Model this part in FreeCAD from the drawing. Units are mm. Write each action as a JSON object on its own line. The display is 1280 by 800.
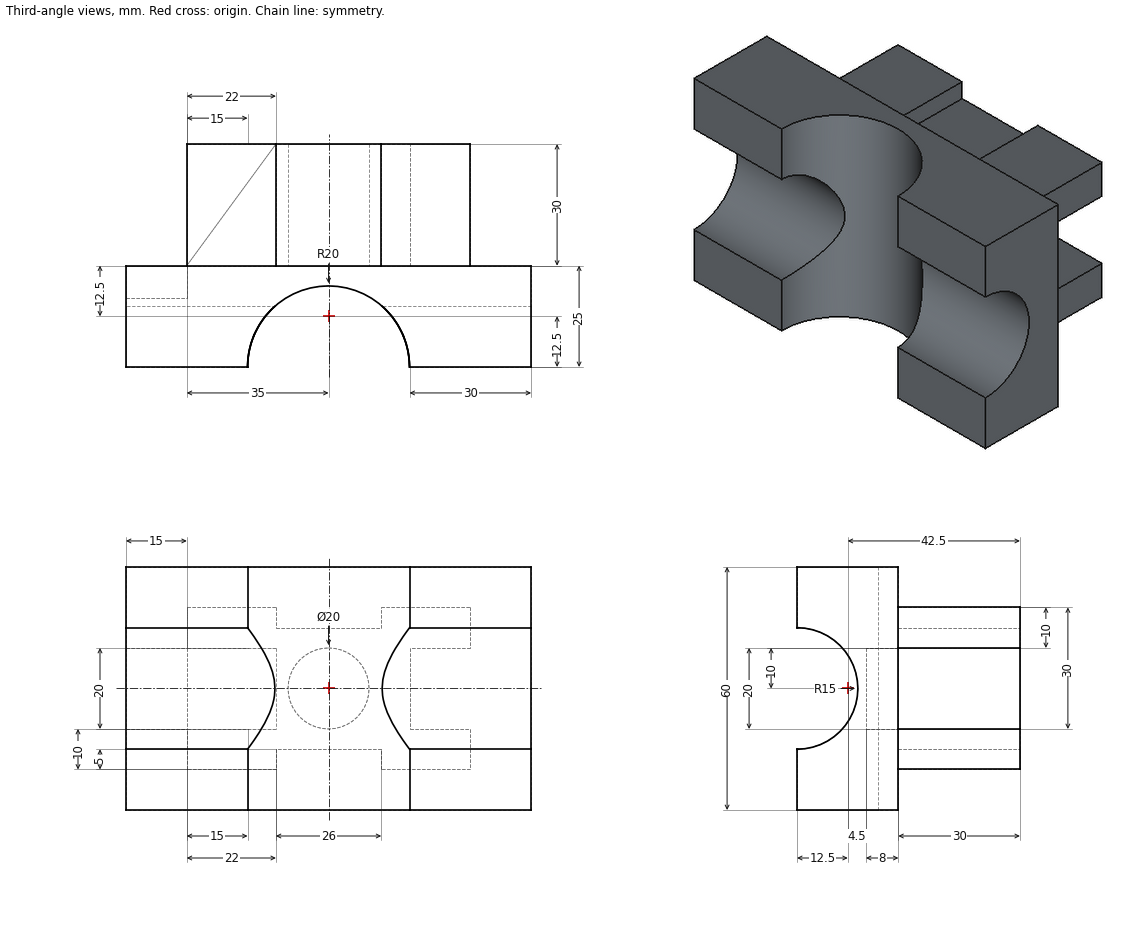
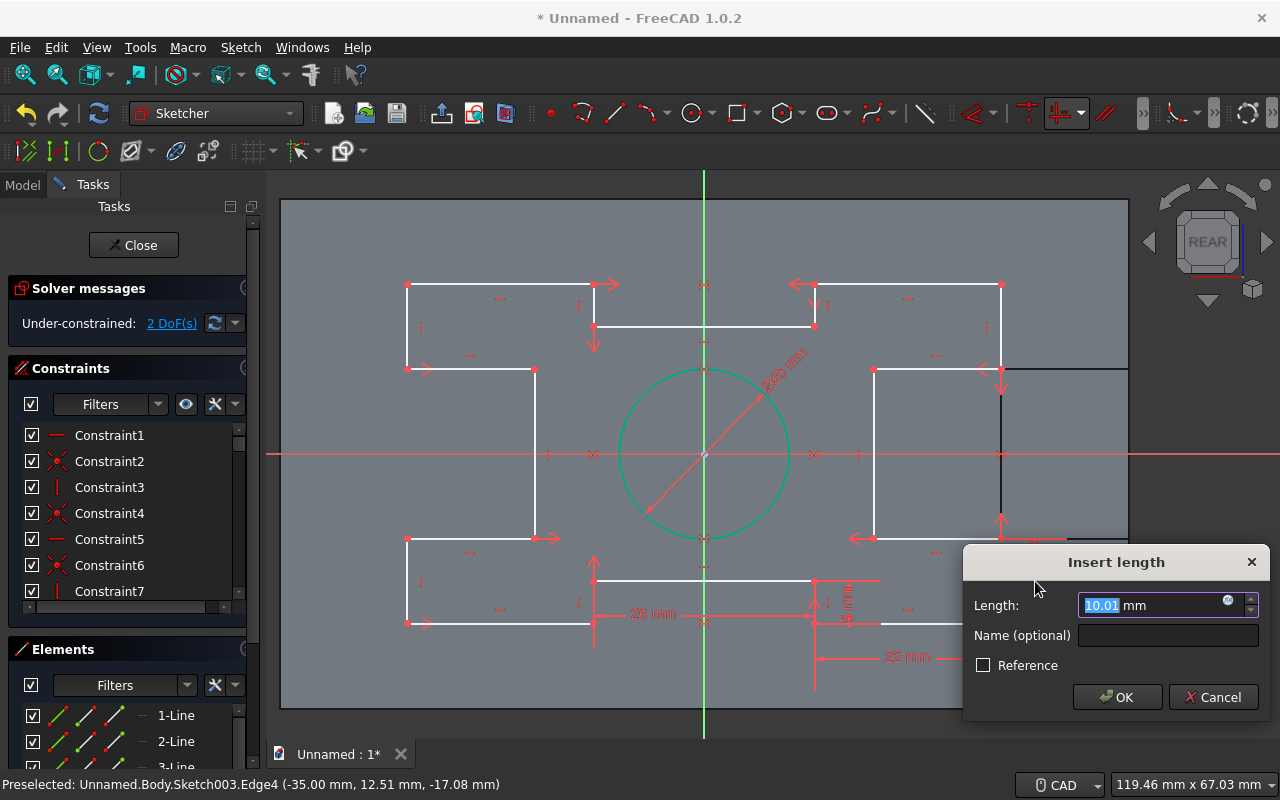
{"action": "type", "text": "10"}
{"action": "key", "text": "Return"}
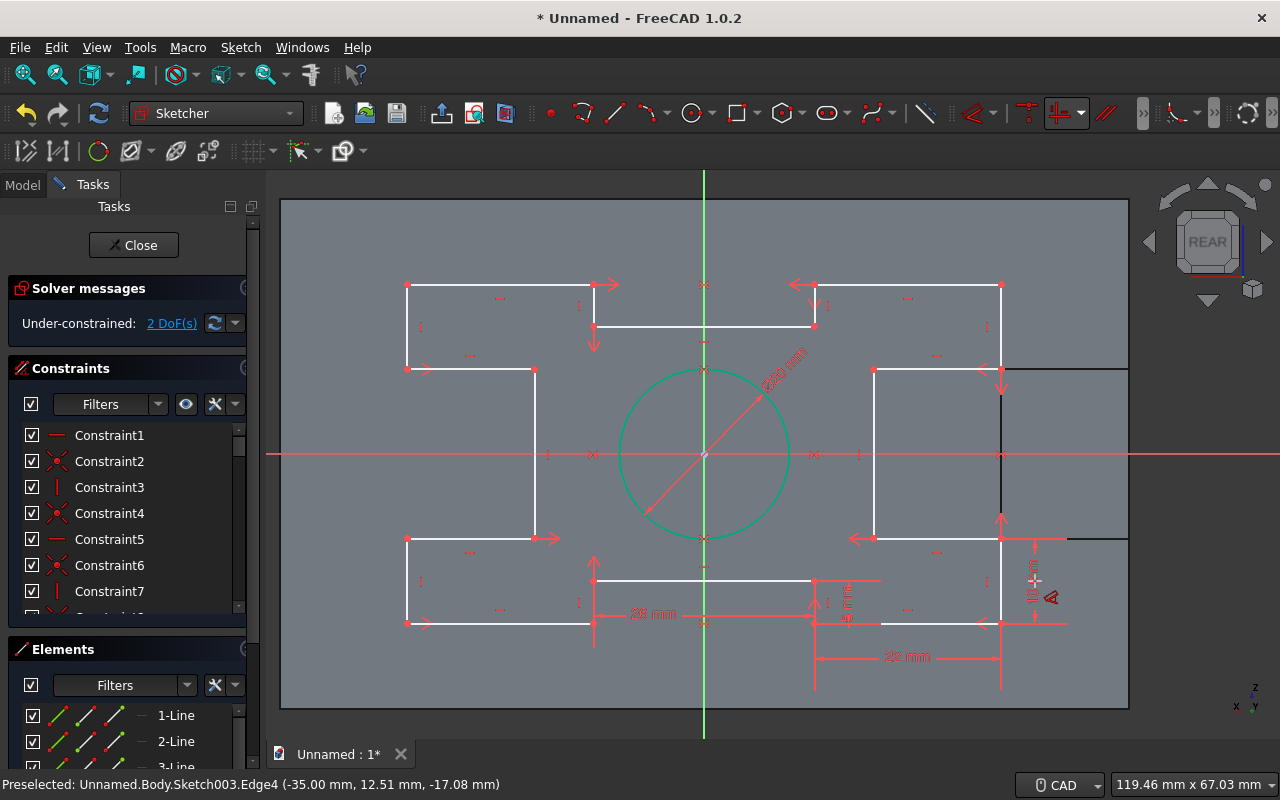
{"action": "left_click", "coordinate": [963, 539]}
{"action": "left_click", "coordinate": [938, 573]}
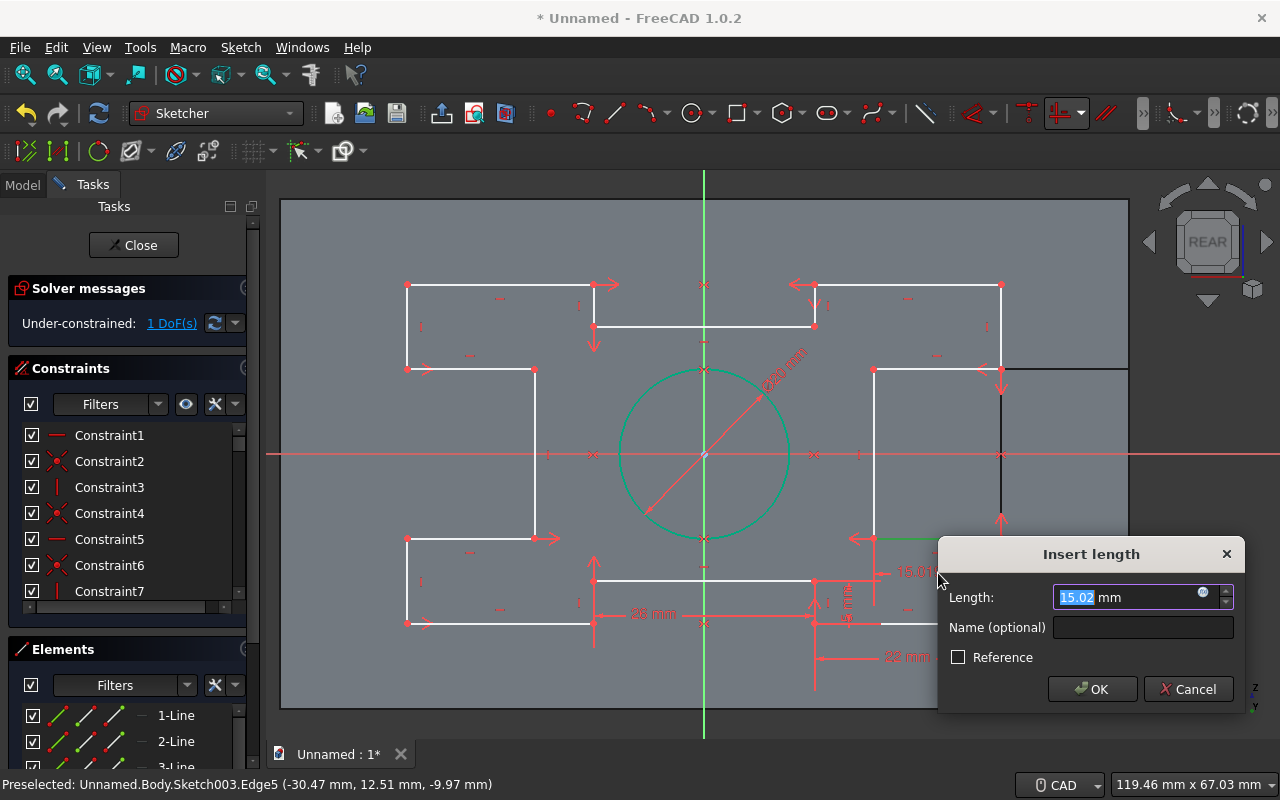
{"action": "type", "text": "15"}
{"action": "key", "text": "Return"}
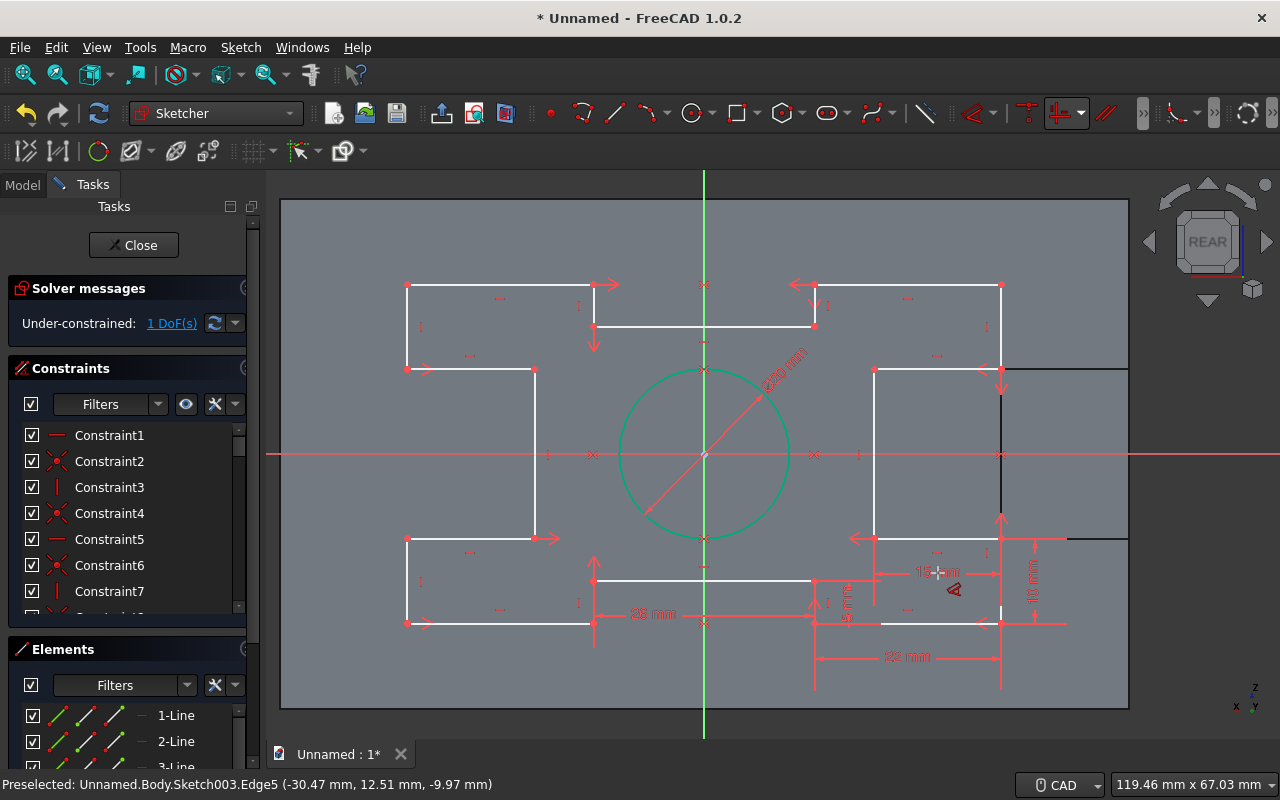
{"action": "left_click", "coordinate": [874, 488]}
{"action": "left_click", "coordinate": [908, 415]}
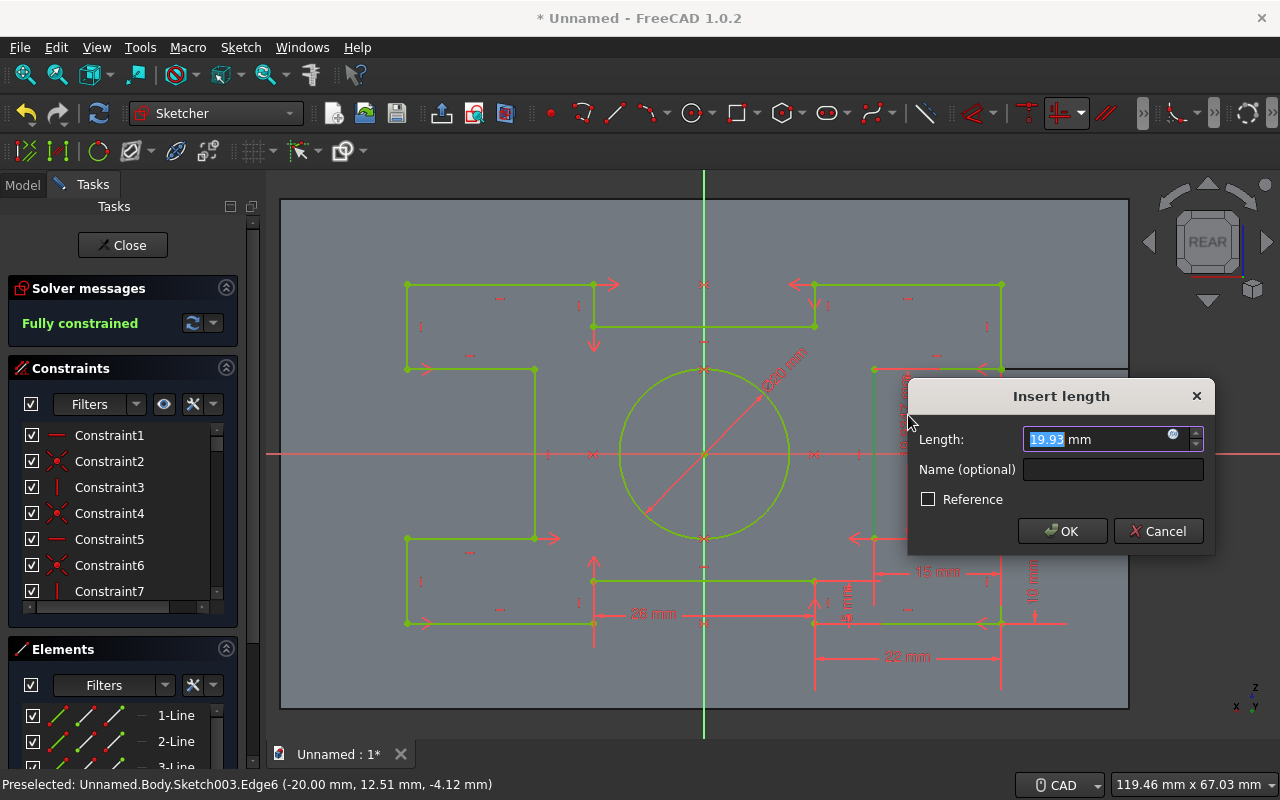
{"action": "type", "text": "20"}
{"action": "key", "text": "Return"}
{"action": "key", "text": "Escape"}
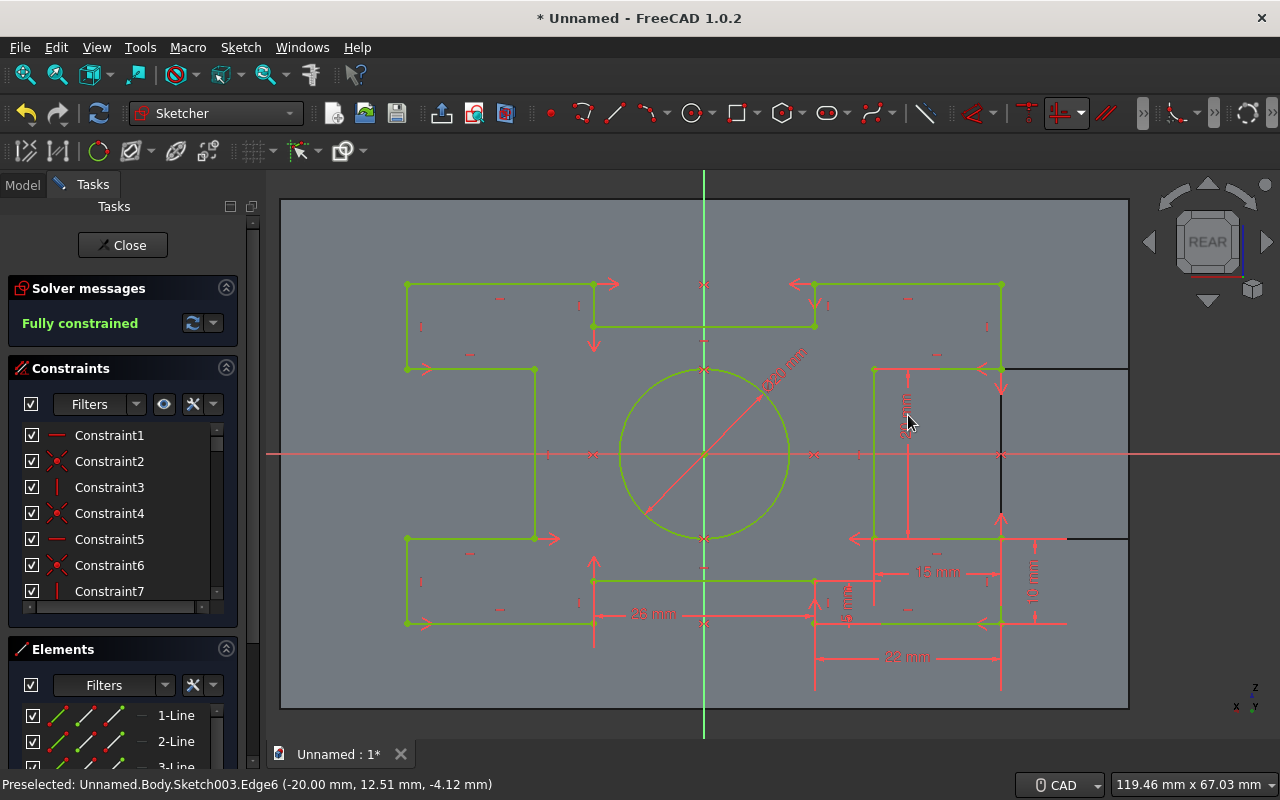
{"action": "left_click", "coordinate": [123, 245]}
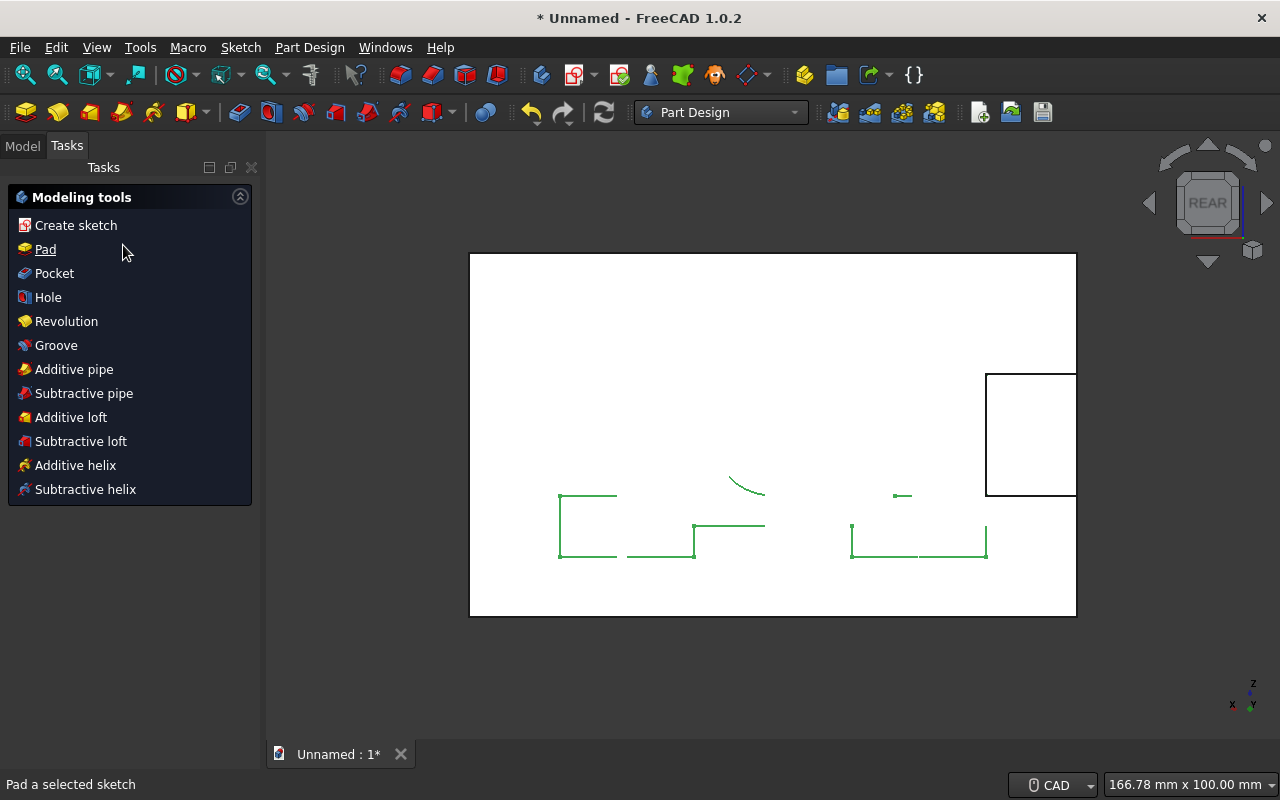
{"action": "left_click", "coordinate": [26, 112]}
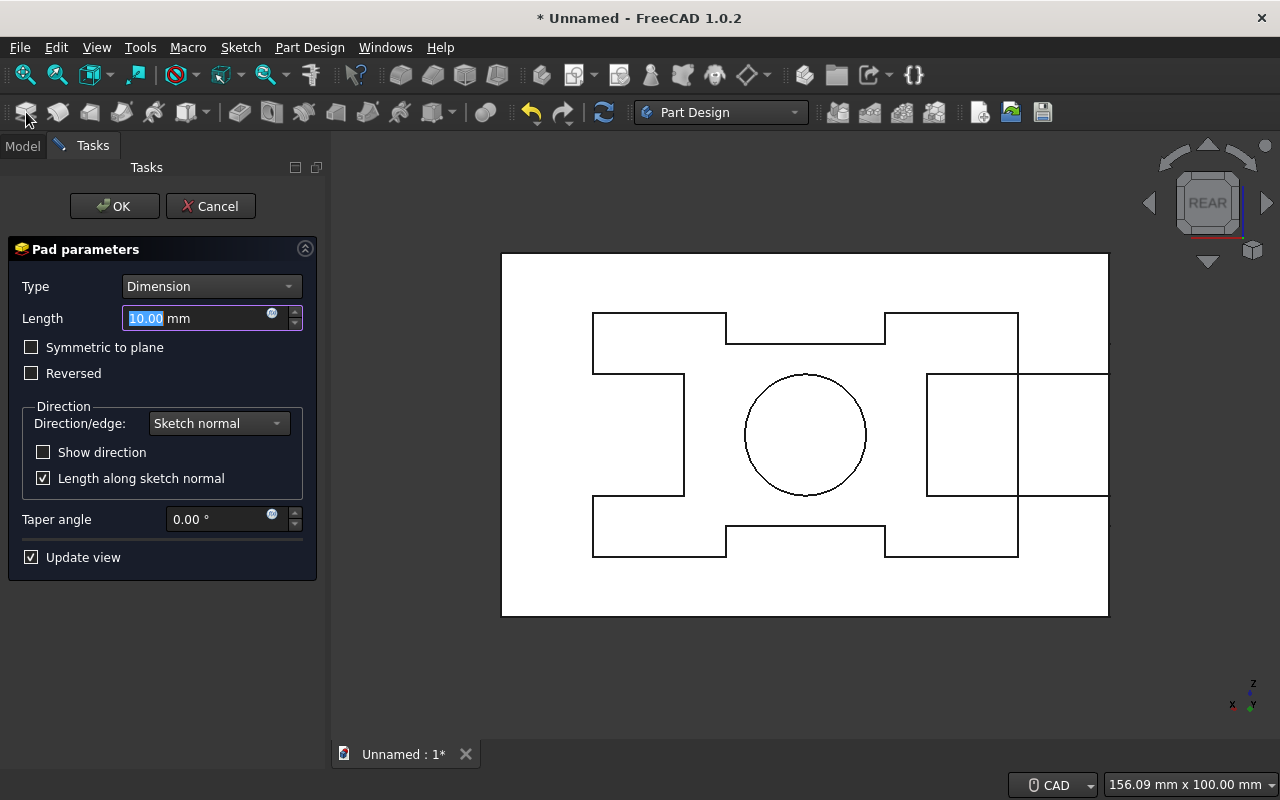
{"action": "type", "text": "30"}
{"action": "key", "text": "Tab"}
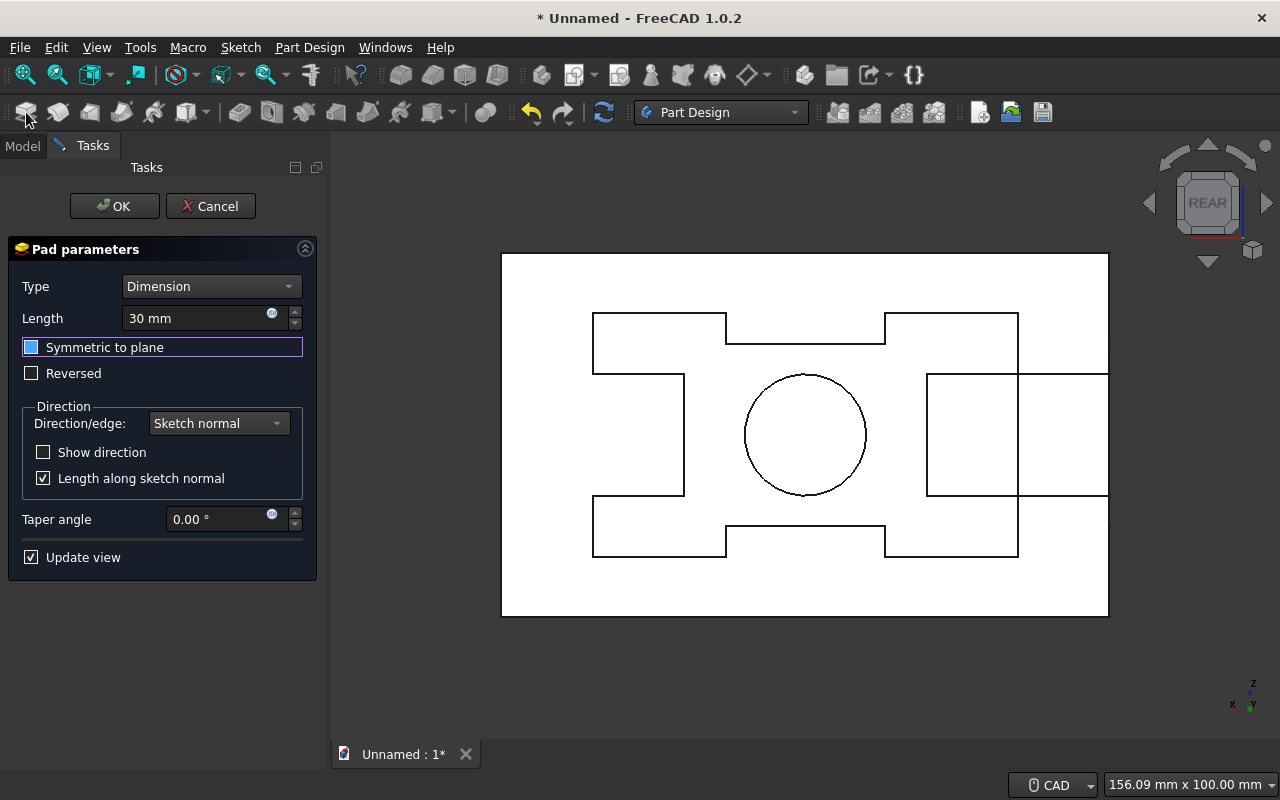
{"action": "left_click", "coordinate": [115, 206]}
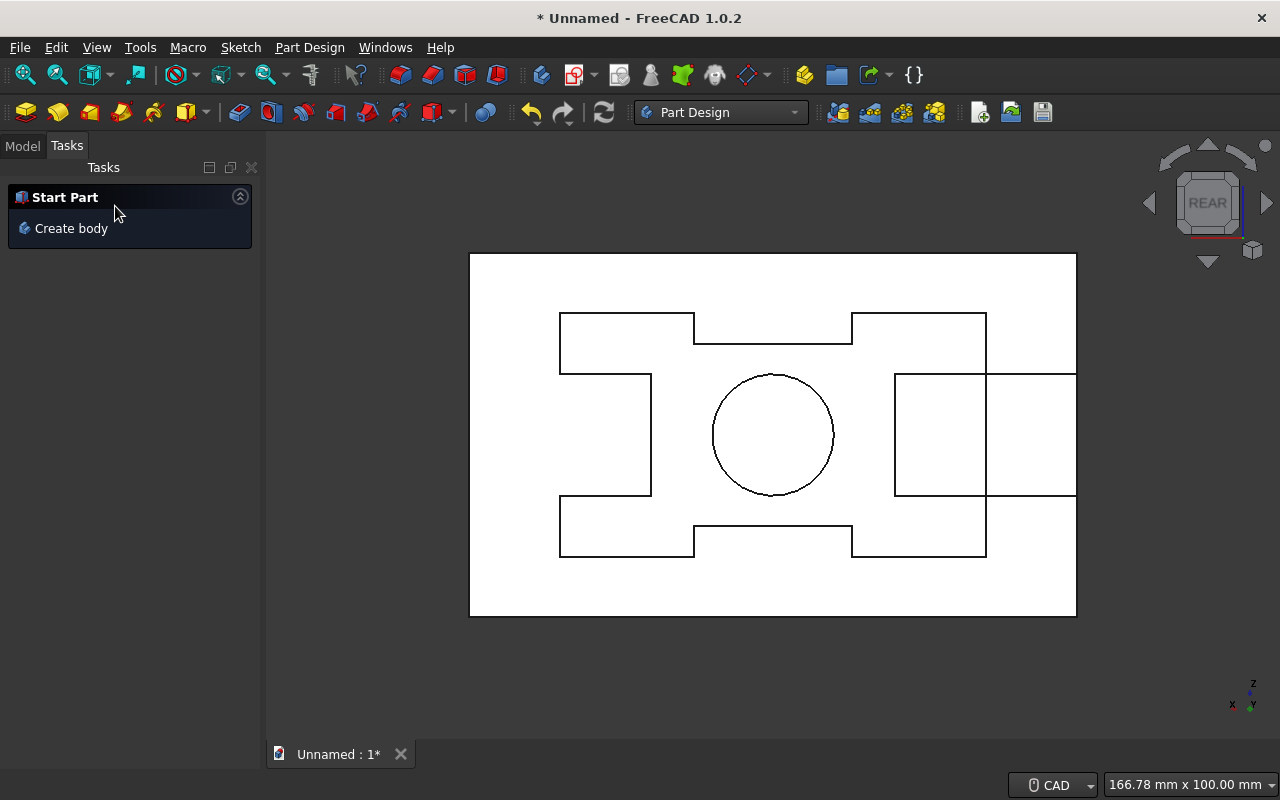
{"action": "key", "text": "6"}